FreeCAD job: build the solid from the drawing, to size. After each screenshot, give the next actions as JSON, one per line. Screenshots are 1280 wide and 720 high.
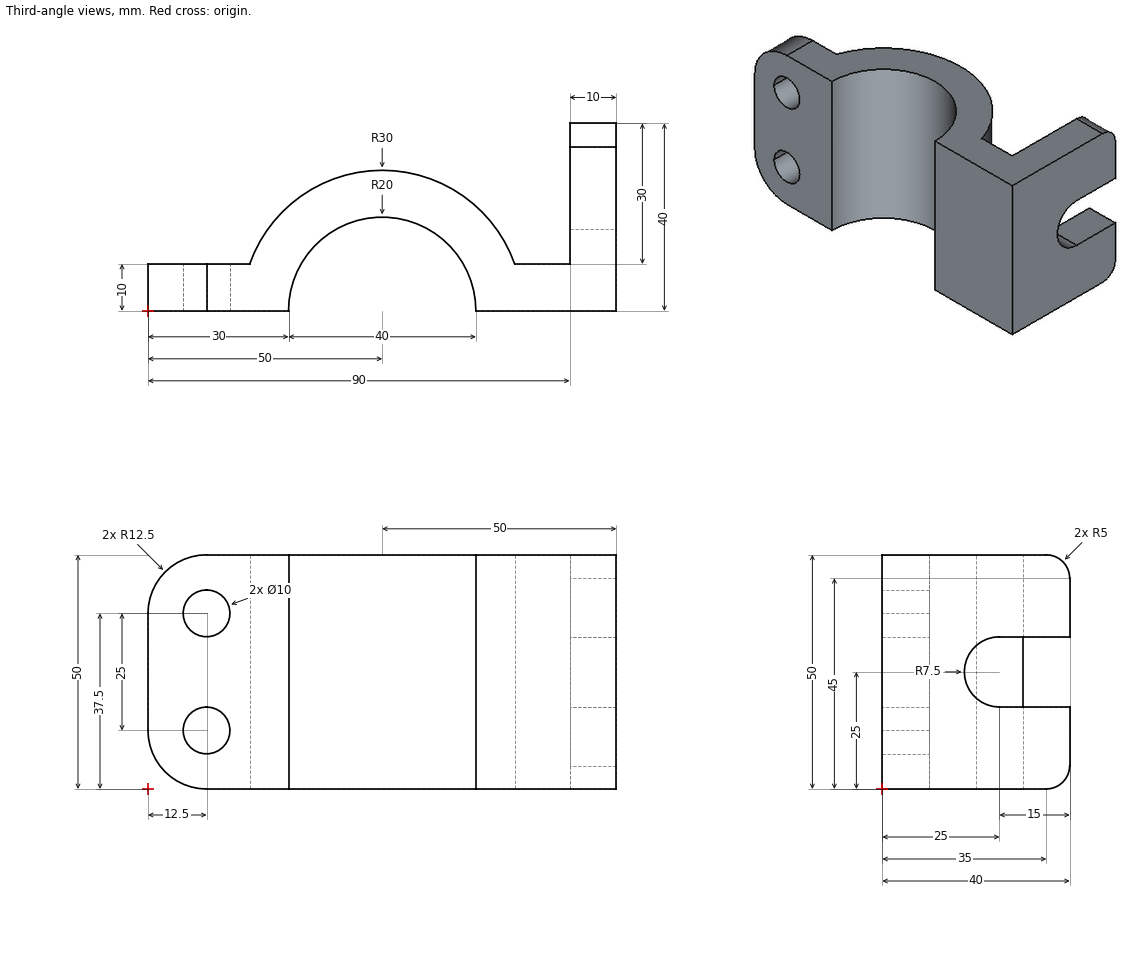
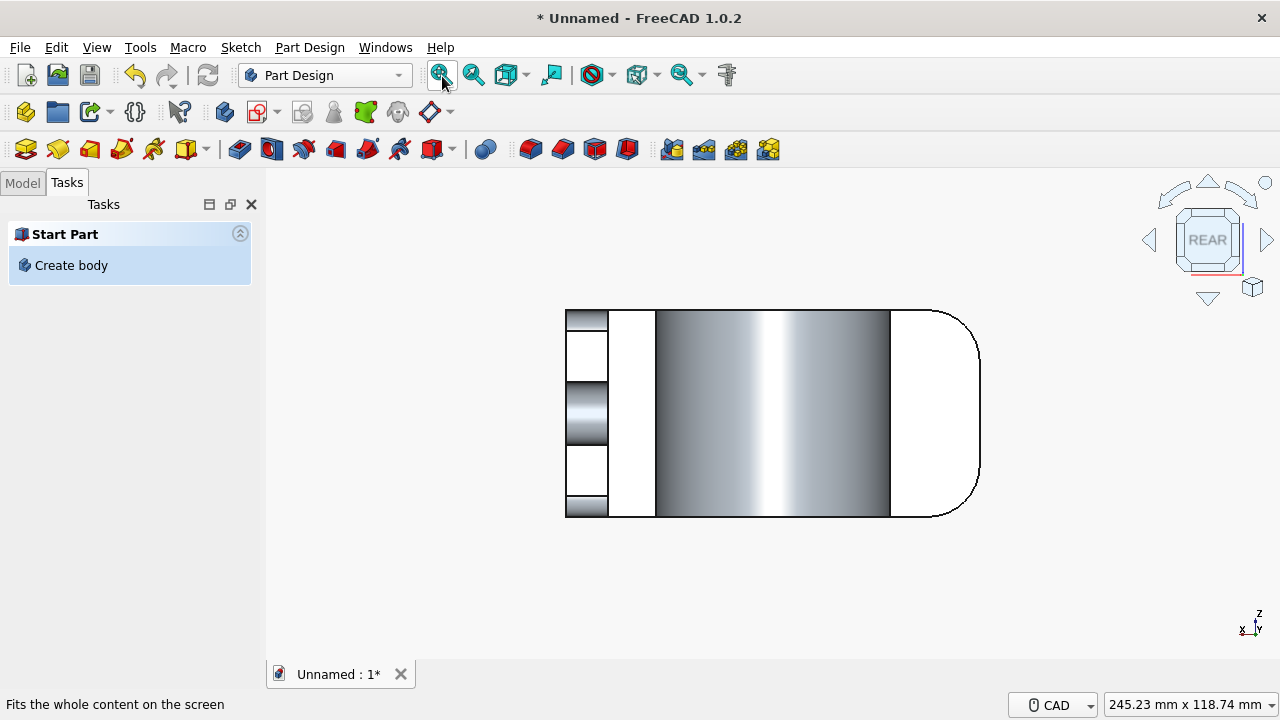
{"action": "left_click", "coordinate": [935, 383]}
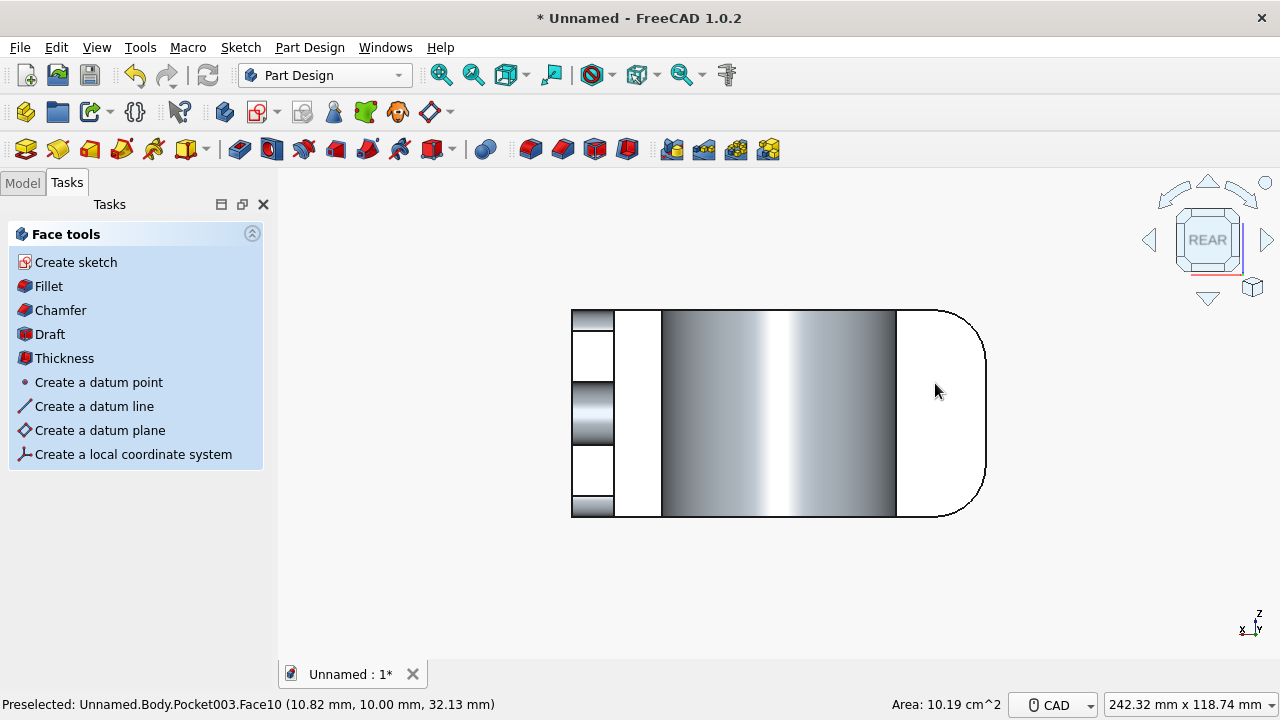
{"action": "left_click", "coordinate": [258, 112]}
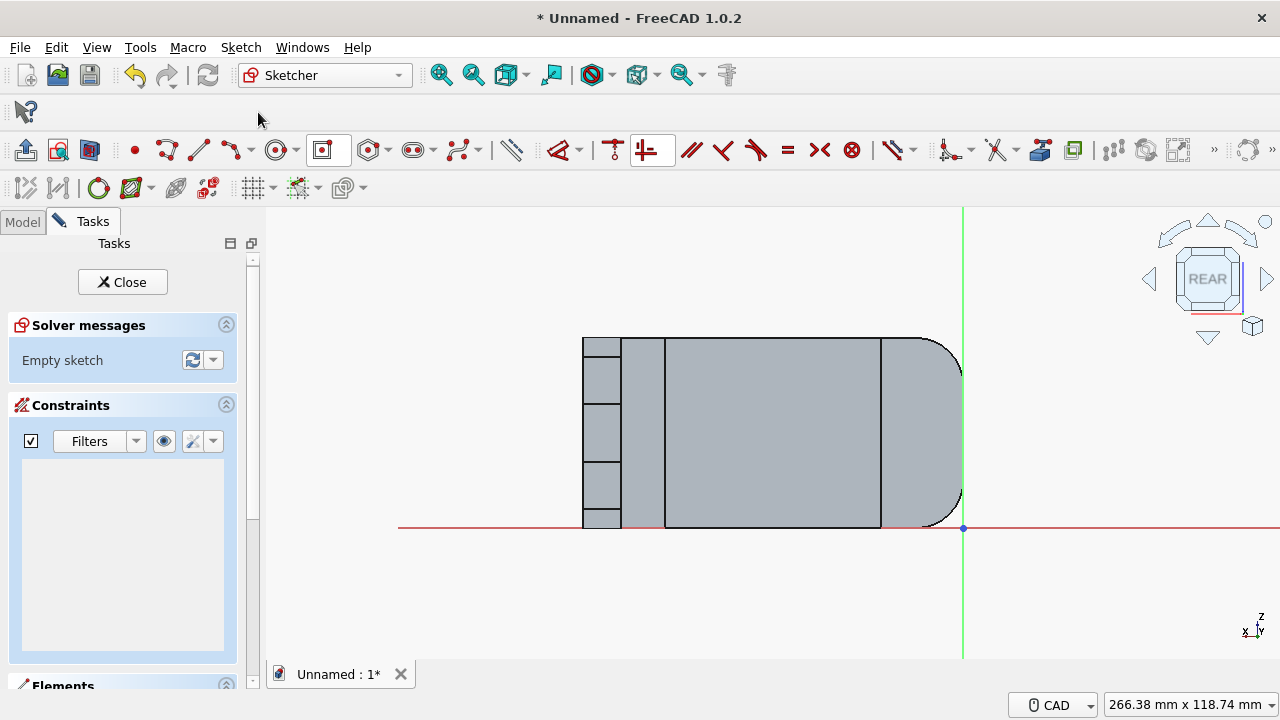
{"action": "scroll", "coordinate": [1115, 465], "scroll_direction": "up", "scroll_amount": 3}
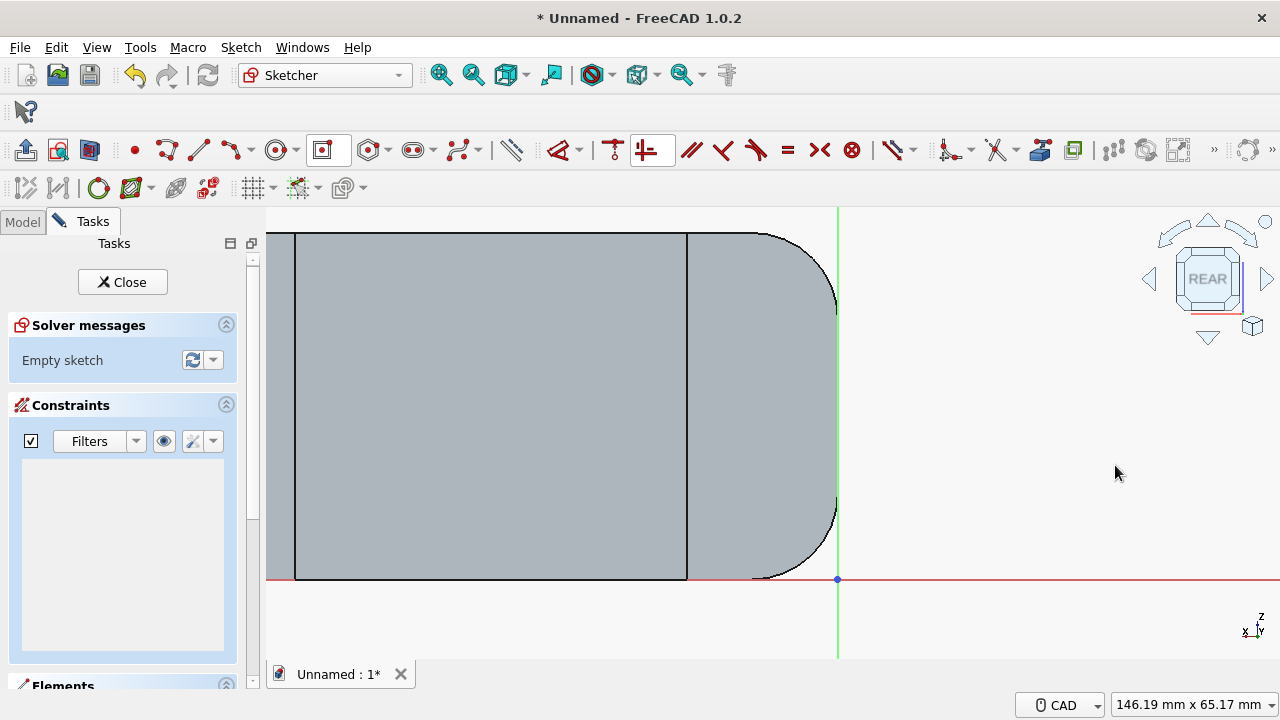
{"action": "left_click", "coordinate": [276, 150]}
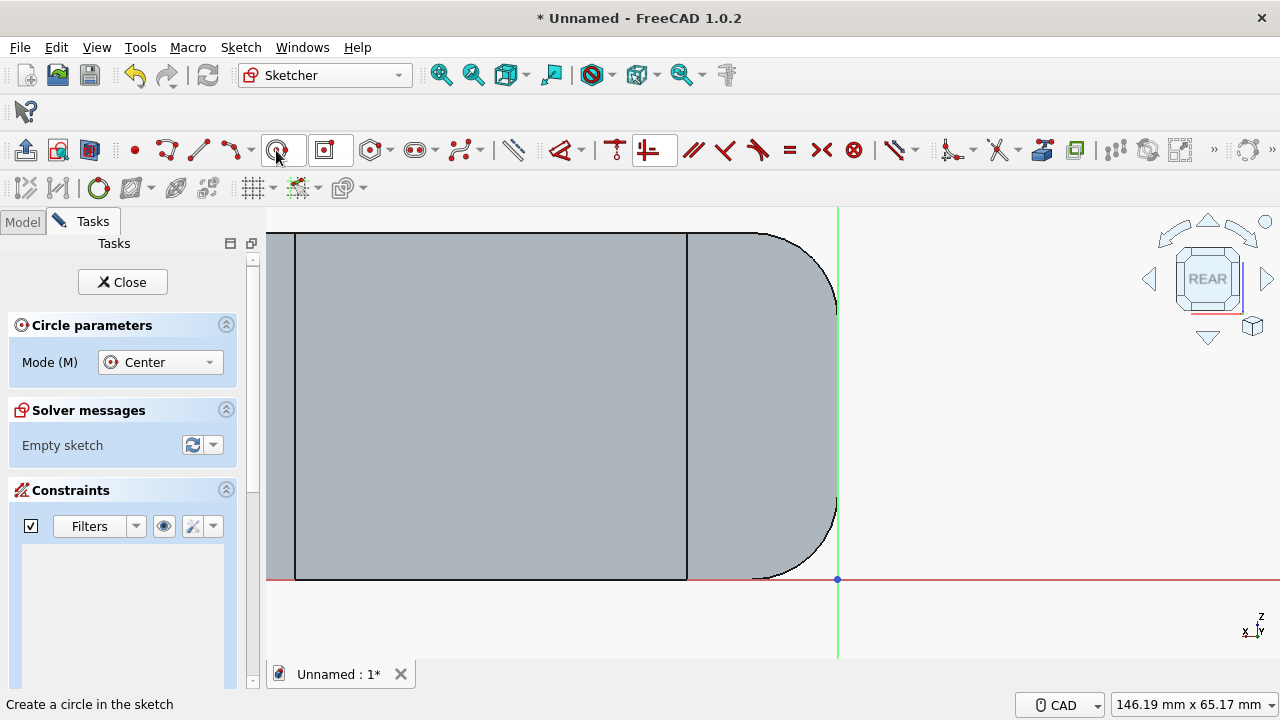
{"action": "left_click", "coordinate": [751, 320]}
{"action": "left_click", "coordinate": [776, 295]}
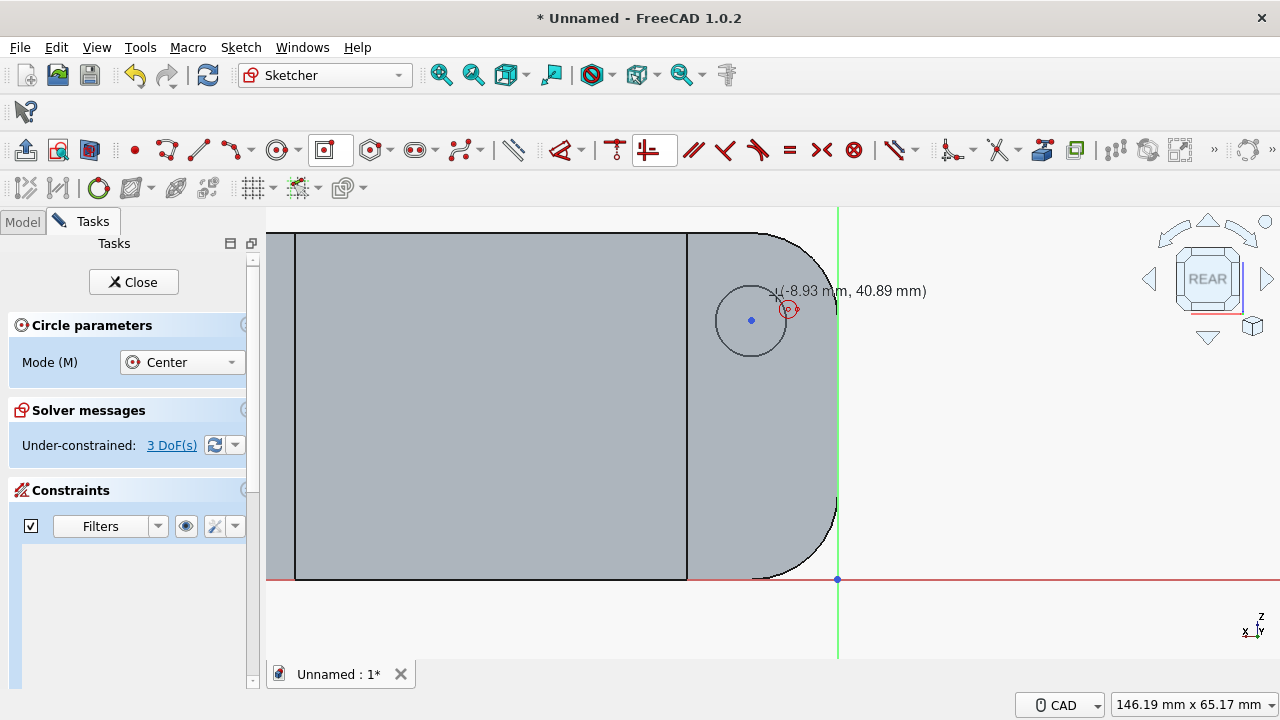
{"action": "left_click", "coordinate": [751, 493]}
{"action": "left_click", "coordinate": [776, 468]}
{"action": "key", "text": "Escape"}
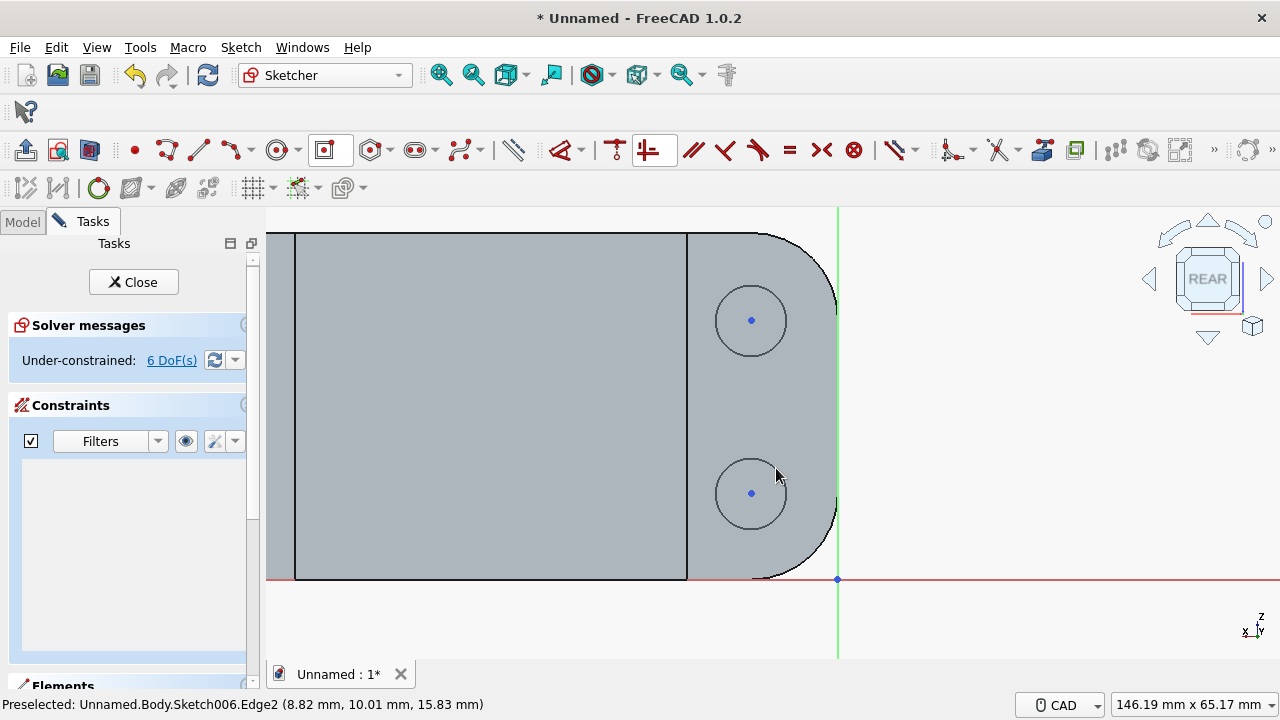
{"action": "left_click", "coordinate": [776, 296]}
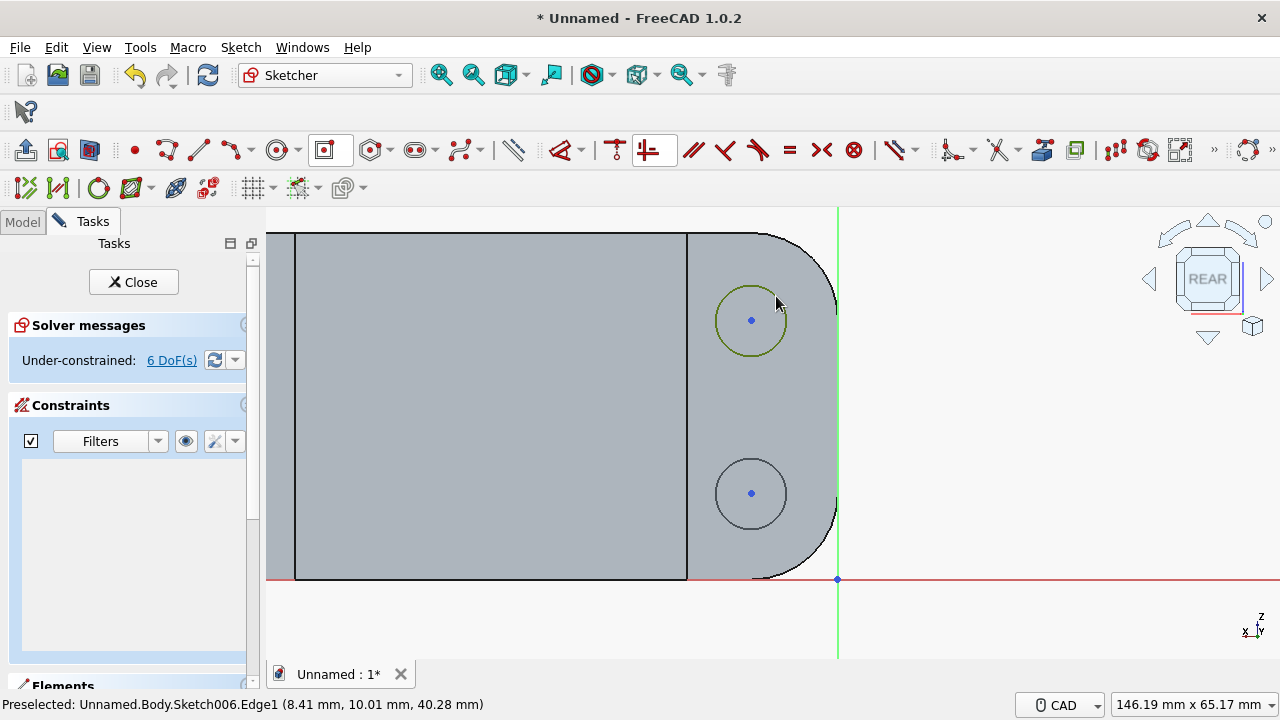
{"action": "left_click", "coordinate": [776, 469]}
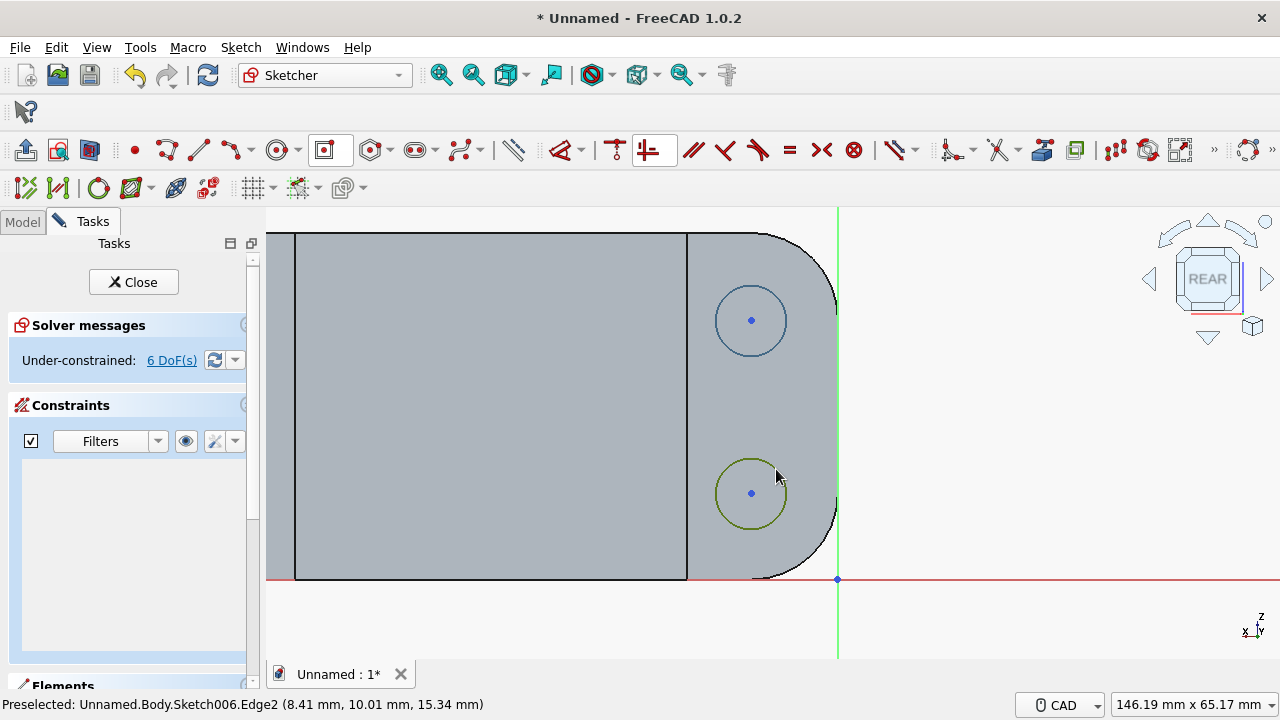
{"action": "left_click", "coordinate": [790, 150]}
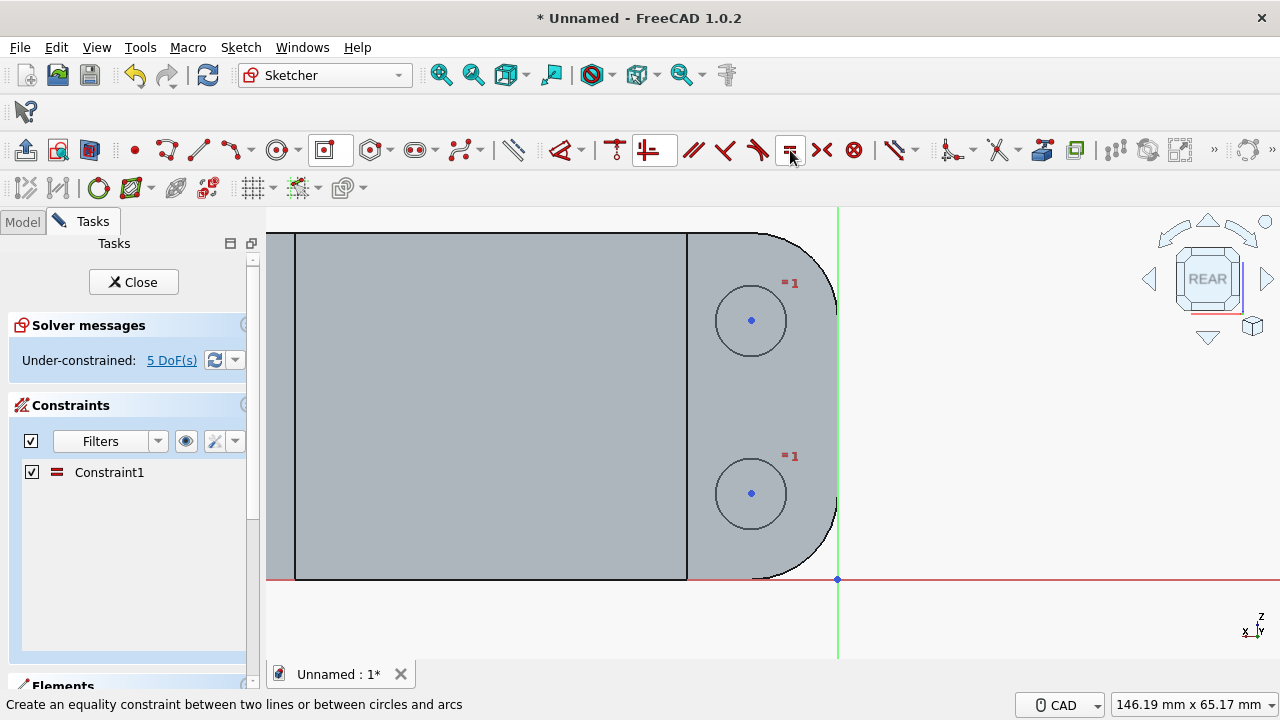
{"action": "left_click", "coordinate": [751, 321]}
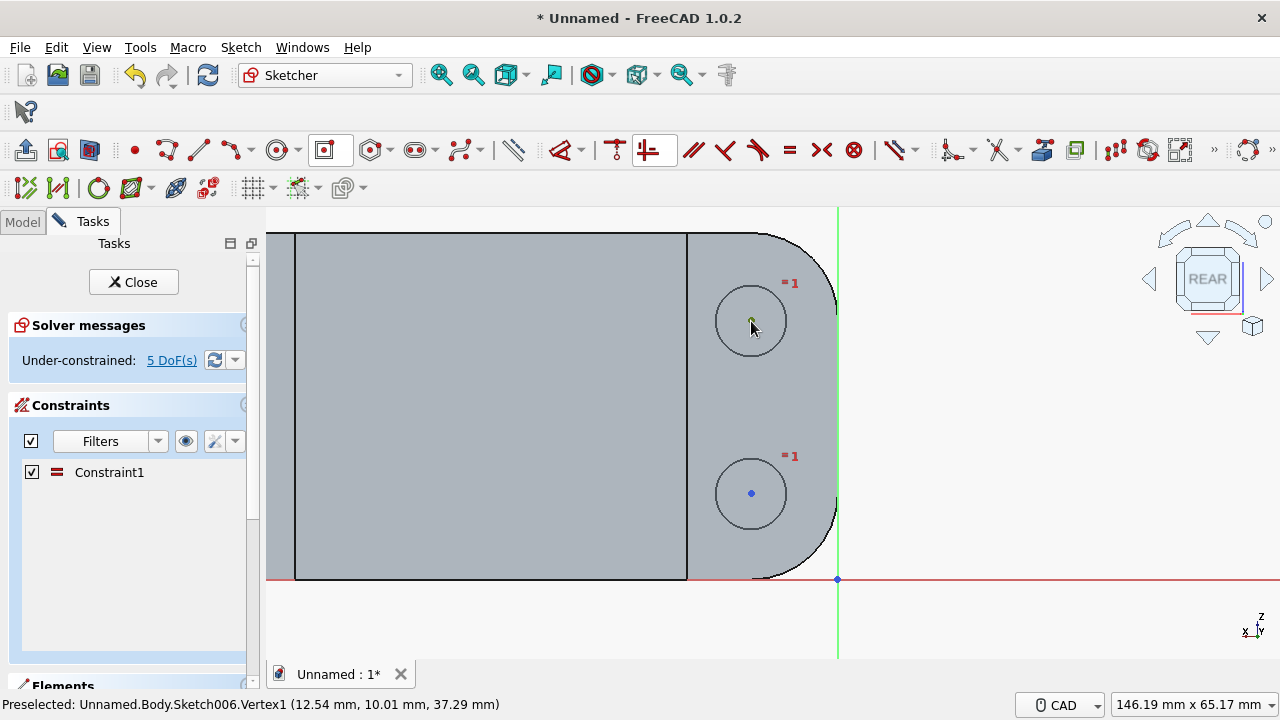
{"action": "left_click", "coordinate": [751, 494]}